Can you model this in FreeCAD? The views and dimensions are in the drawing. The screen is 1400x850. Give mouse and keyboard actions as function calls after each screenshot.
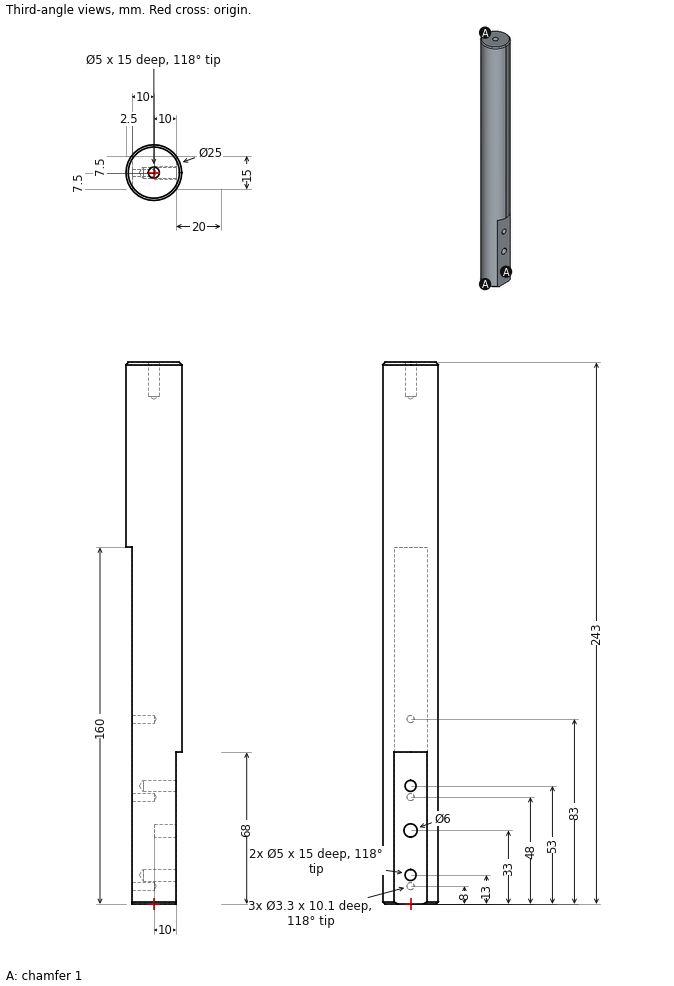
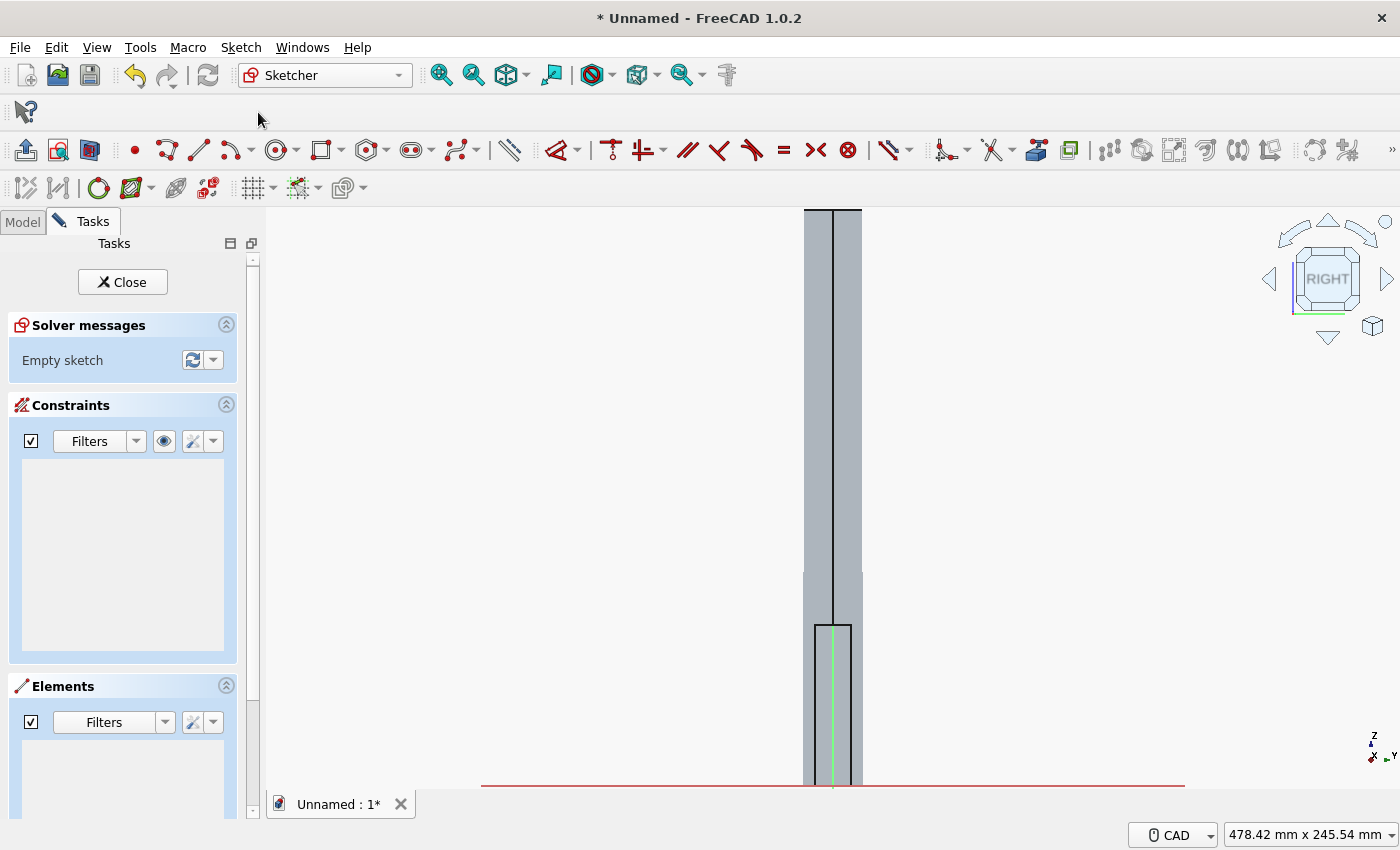
scroll(764, 498, down, 5)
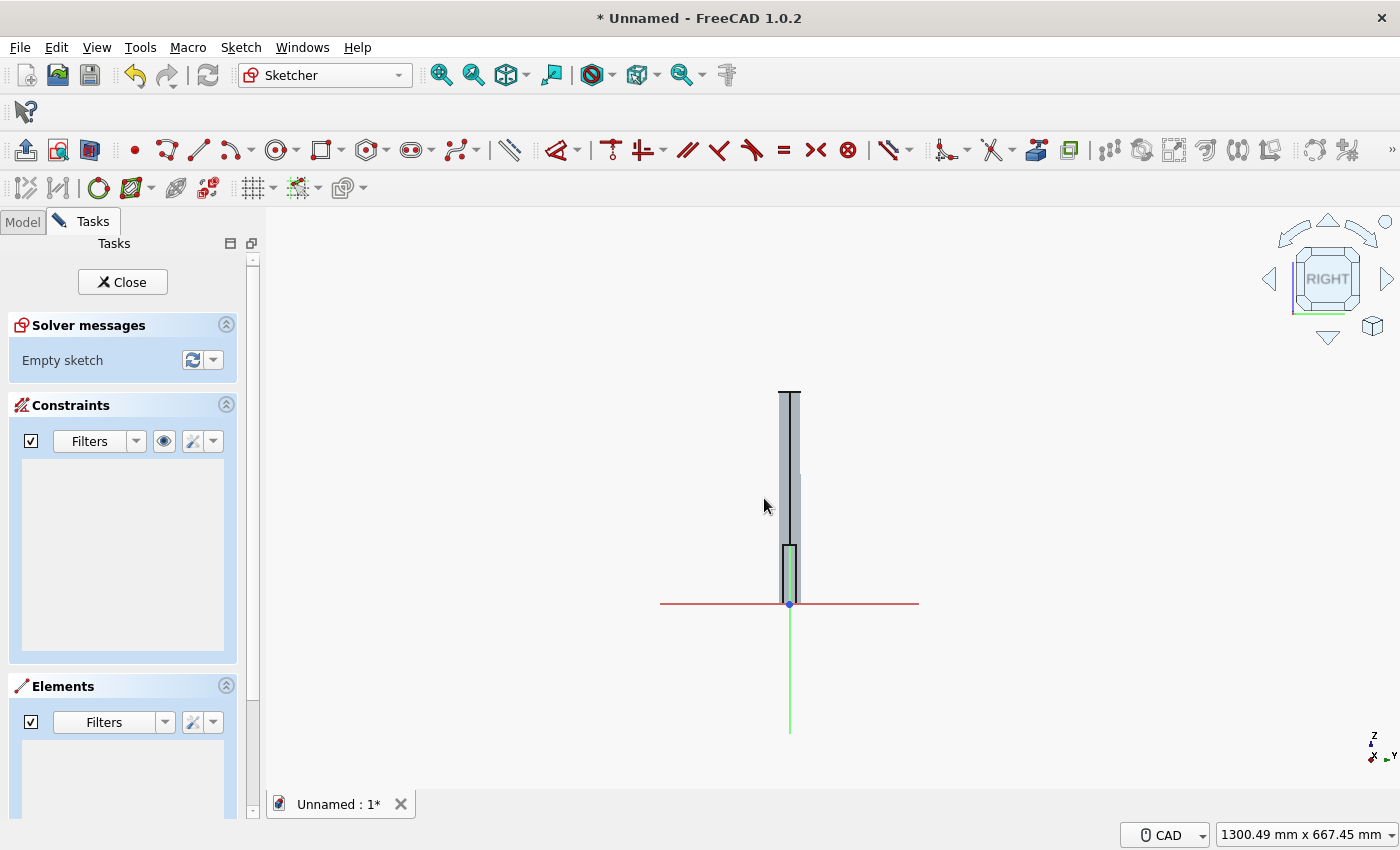
scroll(794, 593, up, 10)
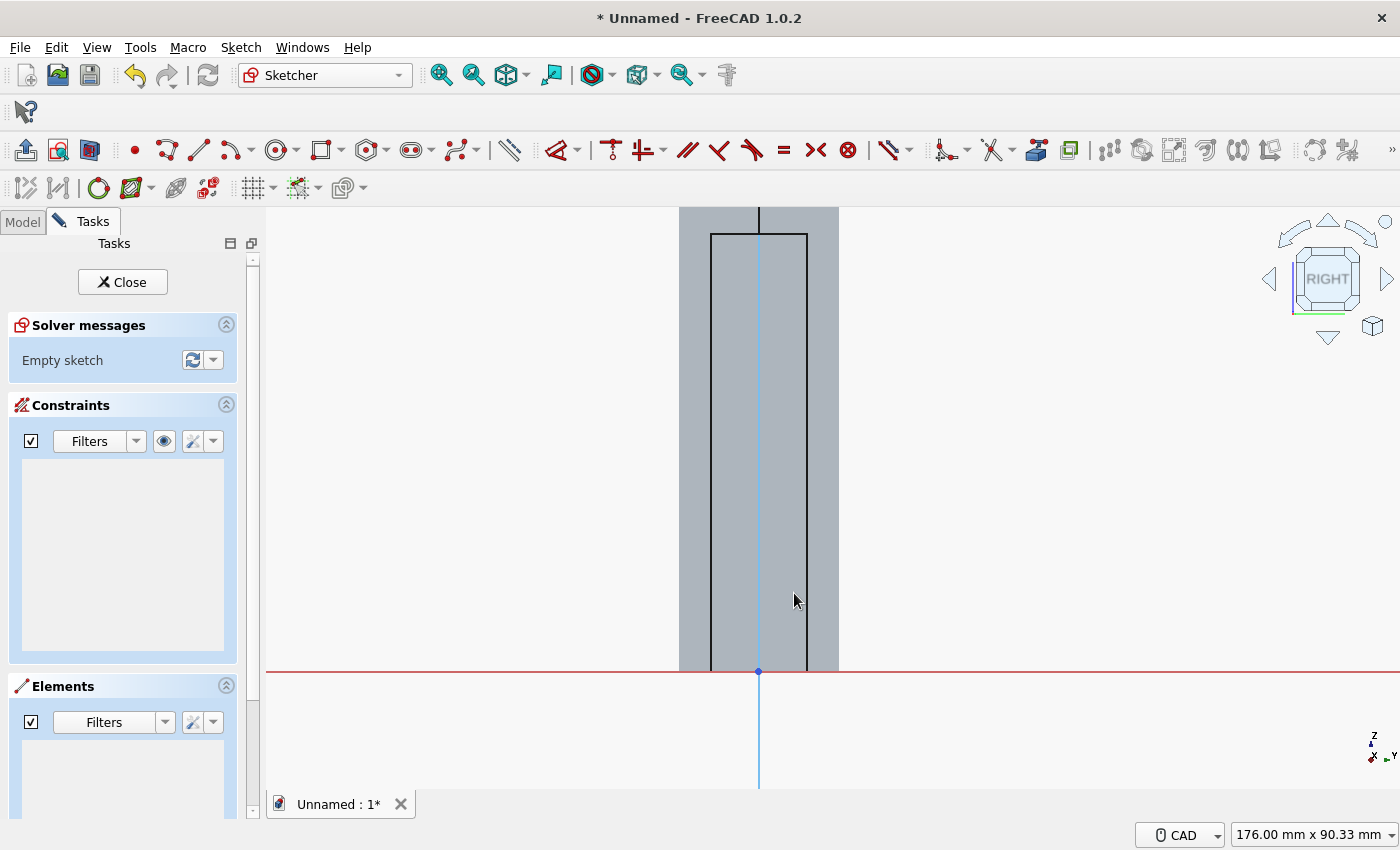
click(276, 150)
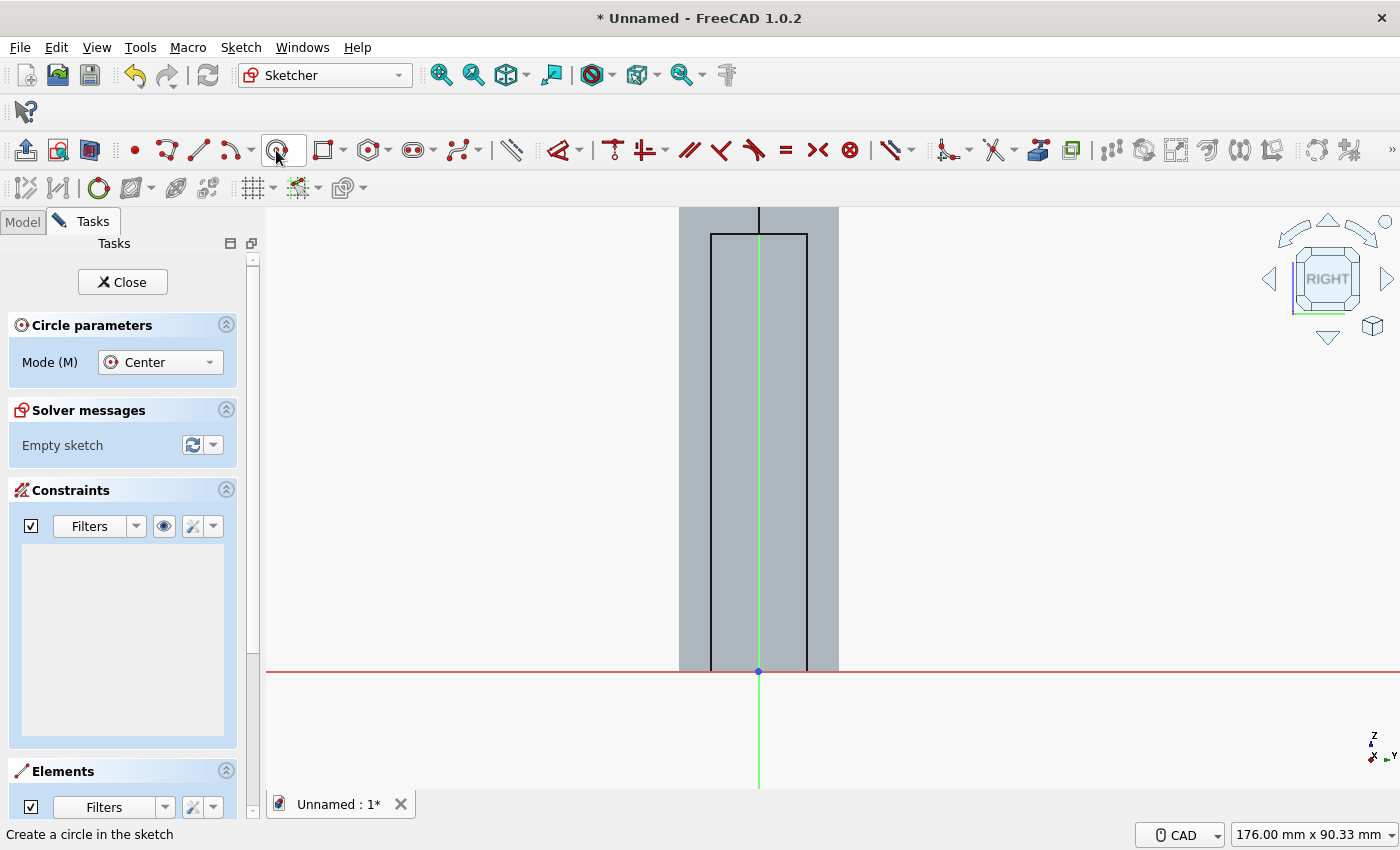
scroll(759, 588, up, 2)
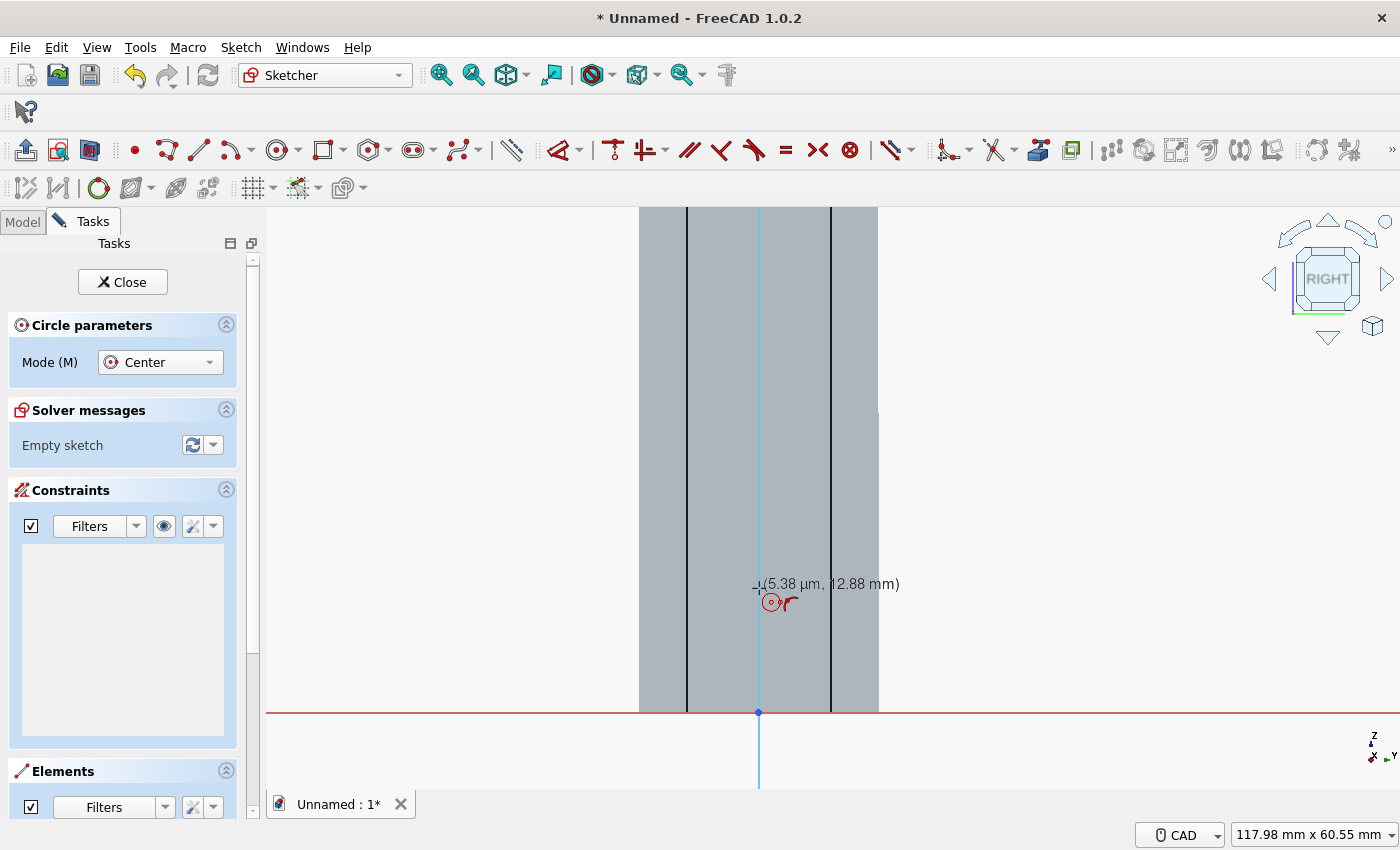
click(759, 588)
click(776, 571)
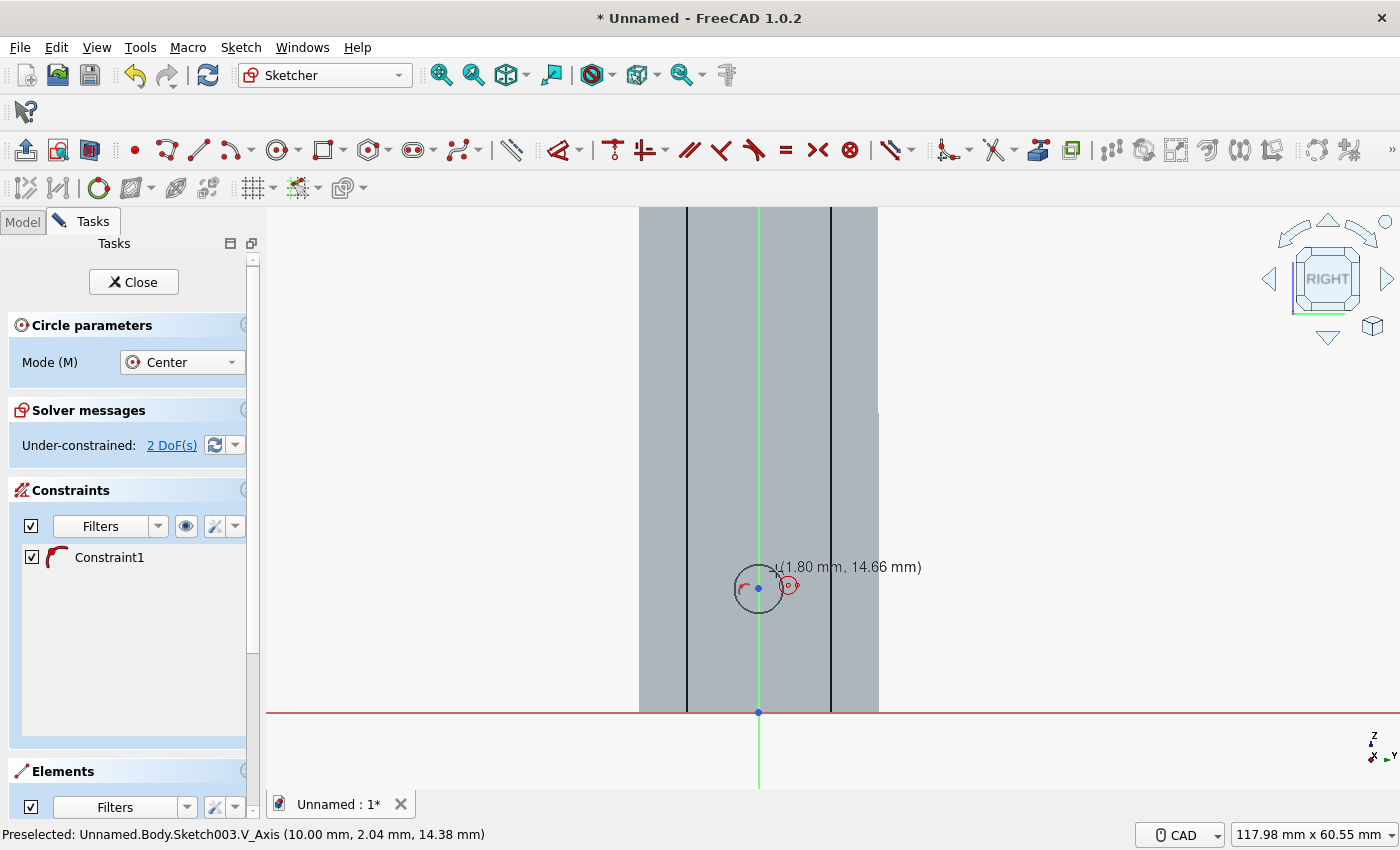
scroll(776, 603, down, 2)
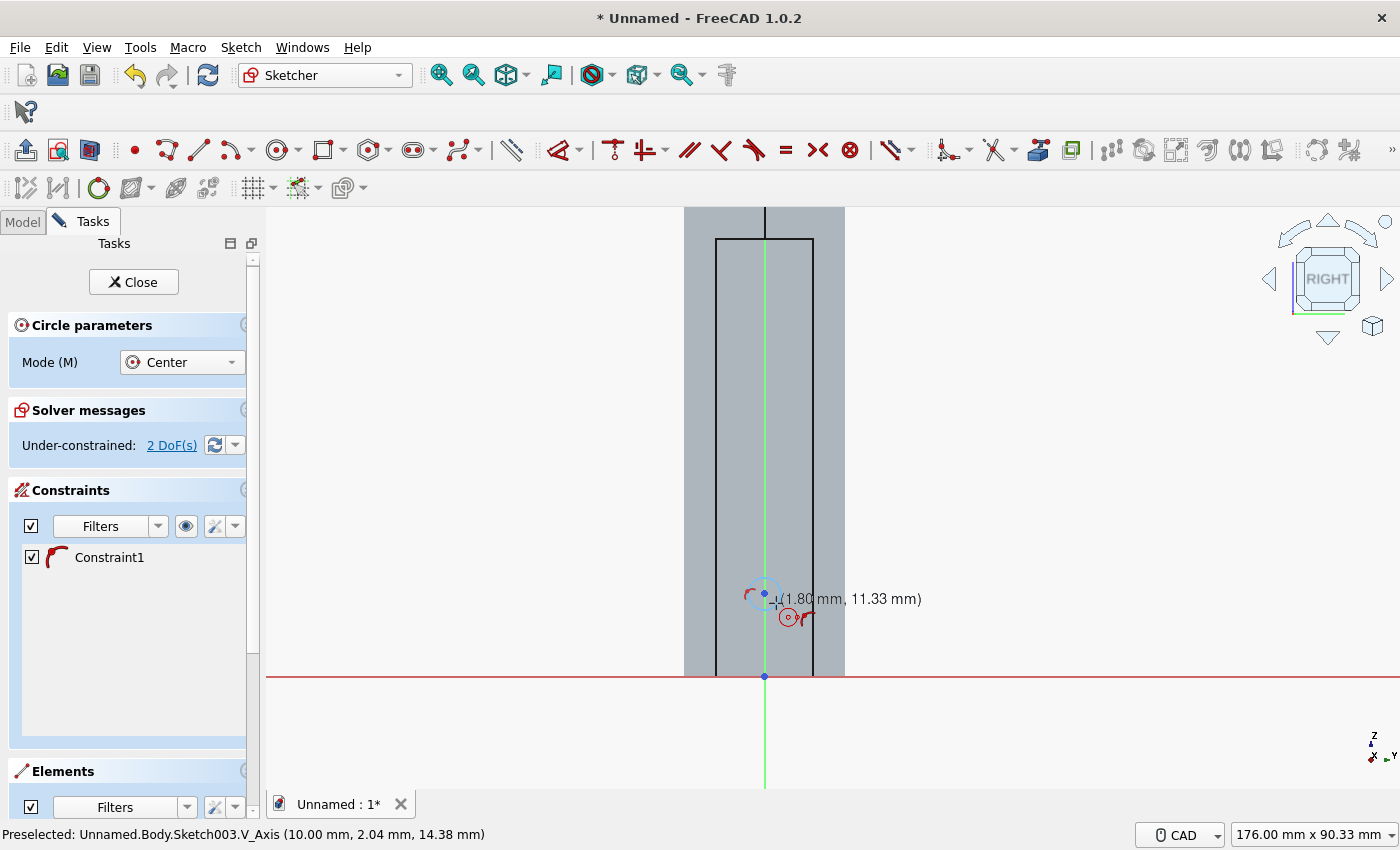
scroll(765, 335, up, 2)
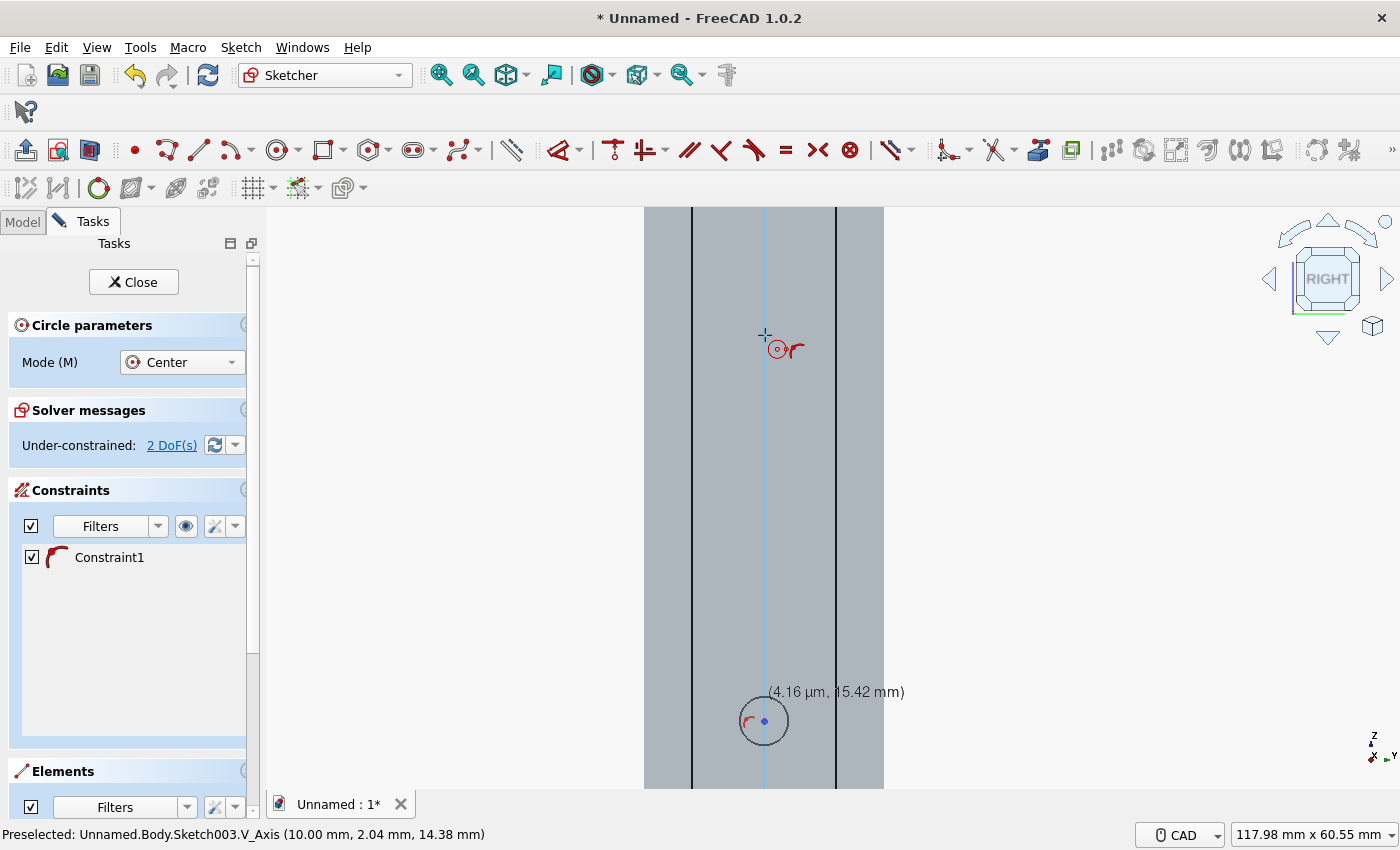
click(764, 336)
click(781, 319)
key(Escape)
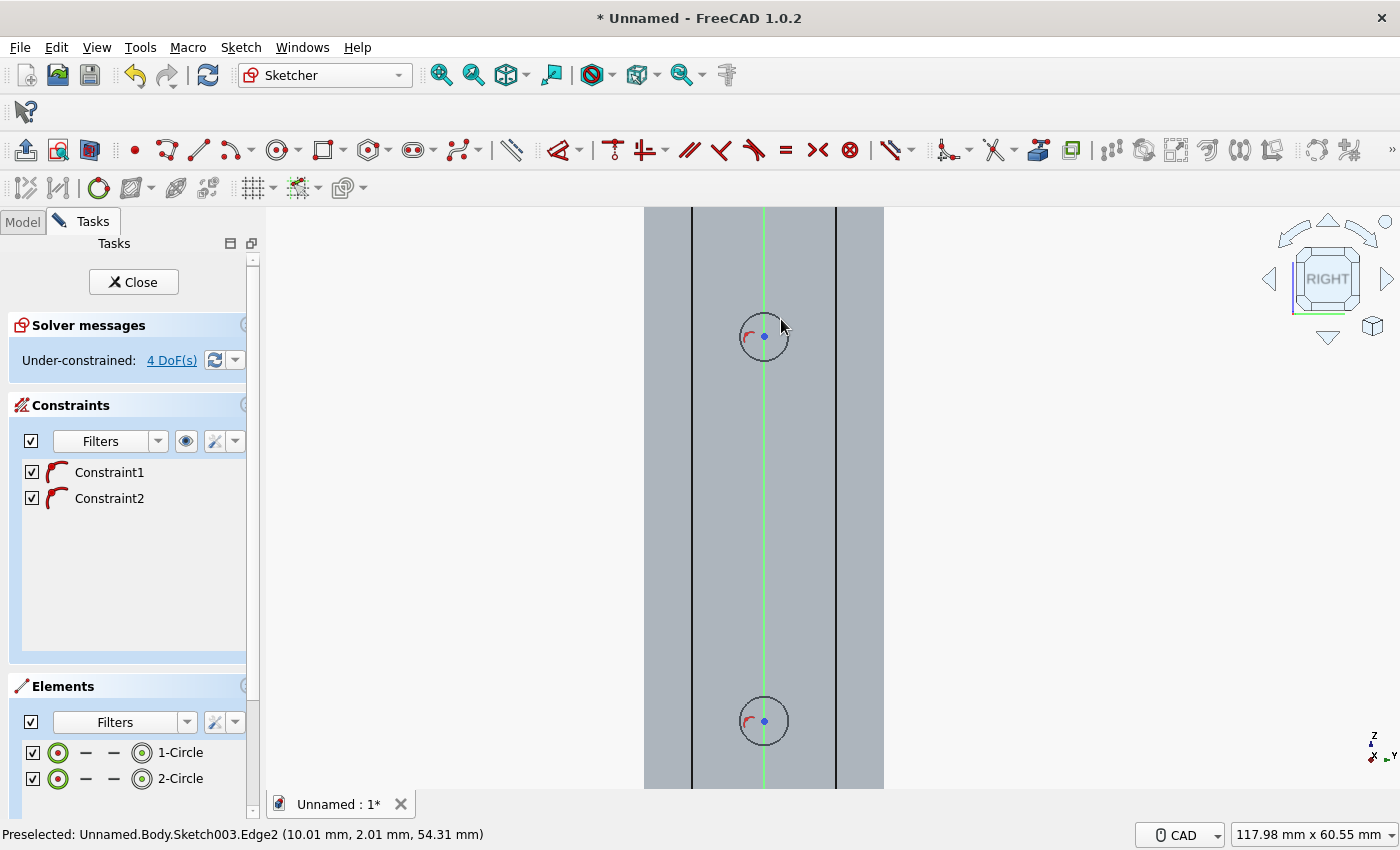
click(781, 704)